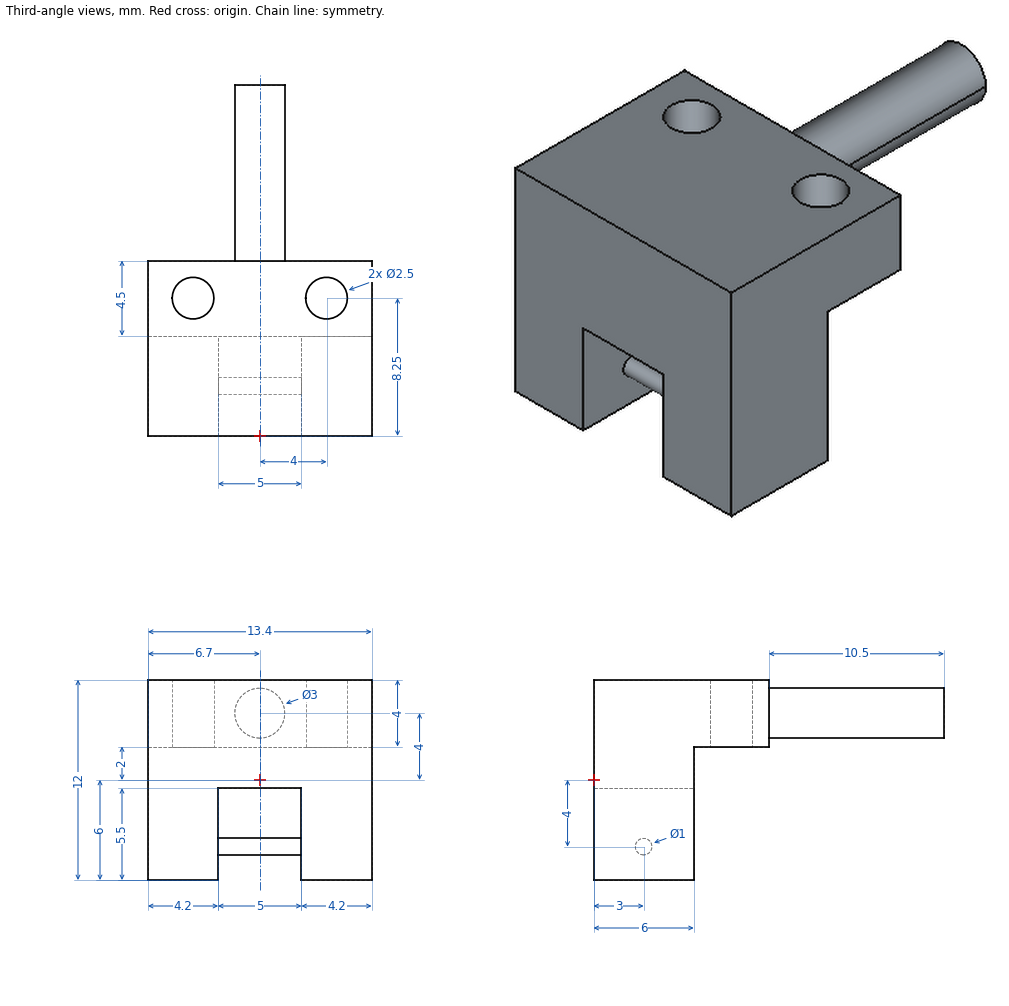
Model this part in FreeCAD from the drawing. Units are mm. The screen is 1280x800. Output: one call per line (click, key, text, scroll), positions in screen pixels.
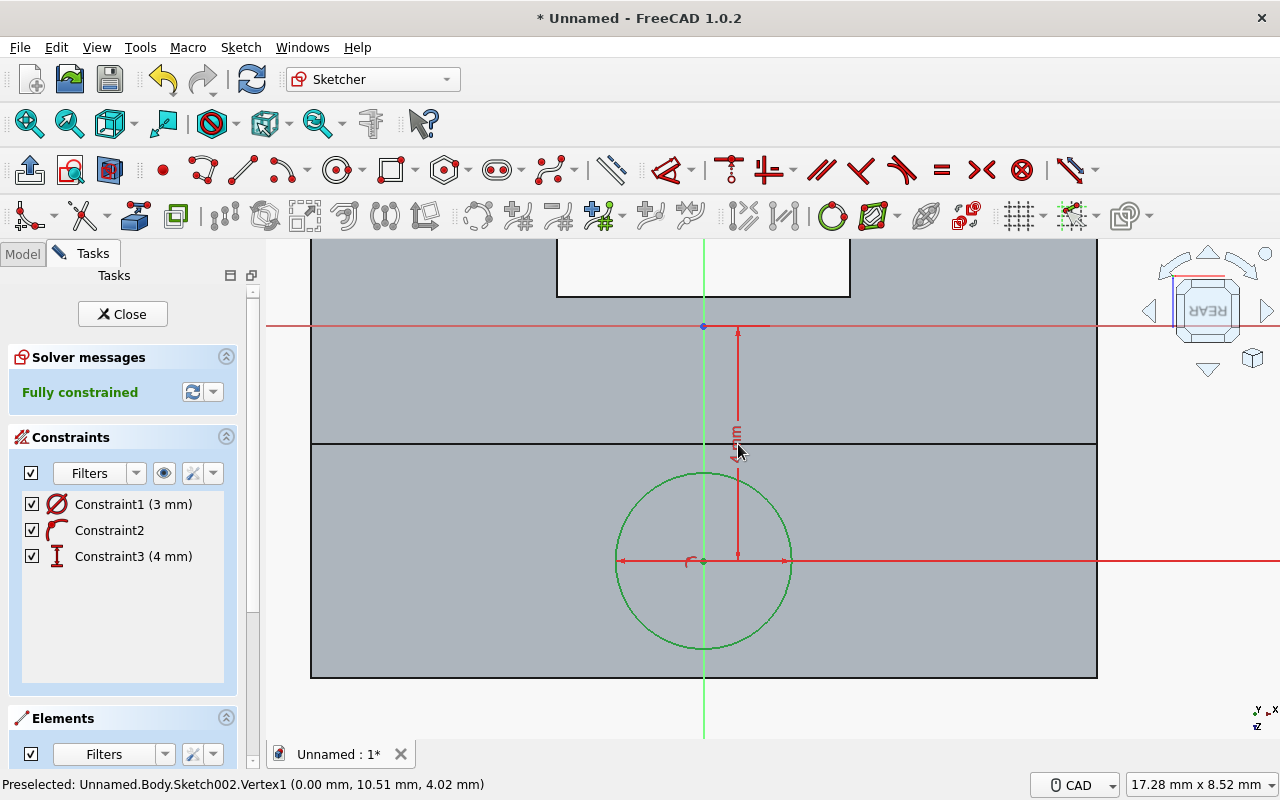
click(123, 314)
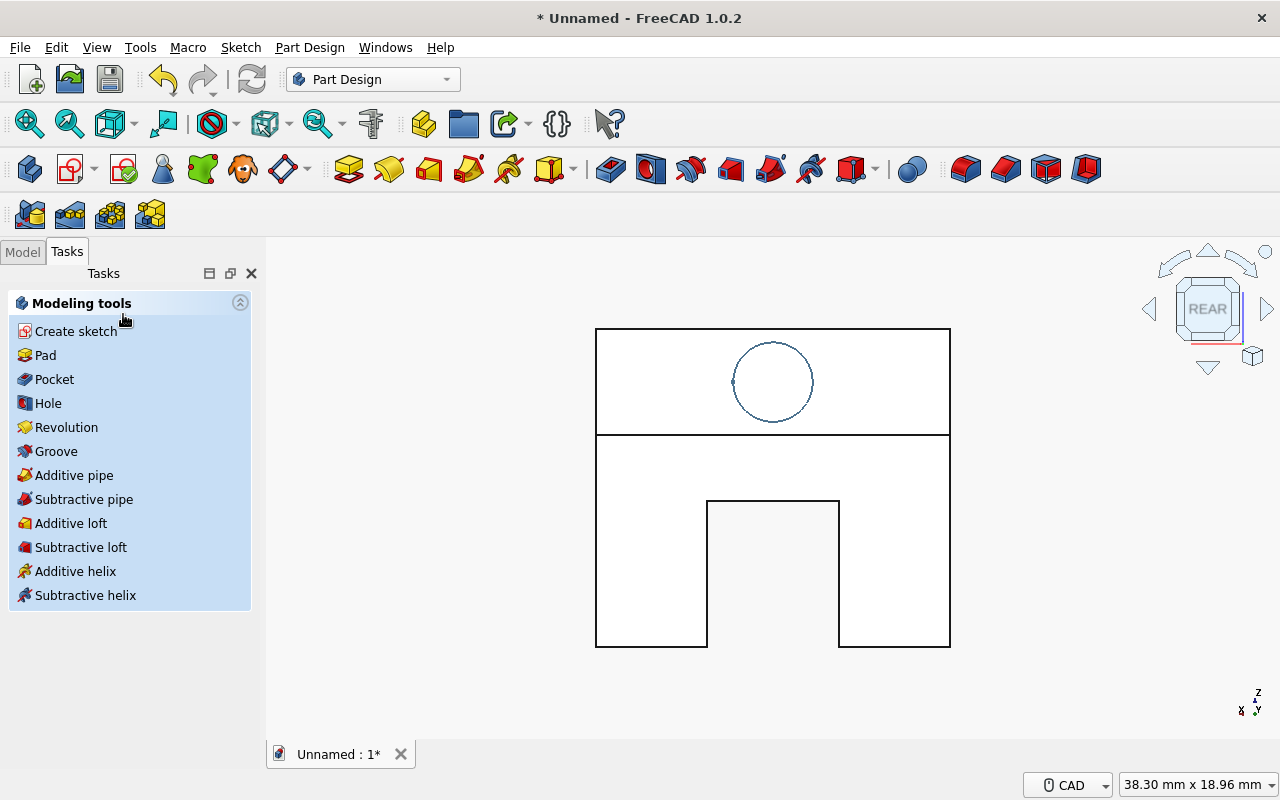
click(350, 170)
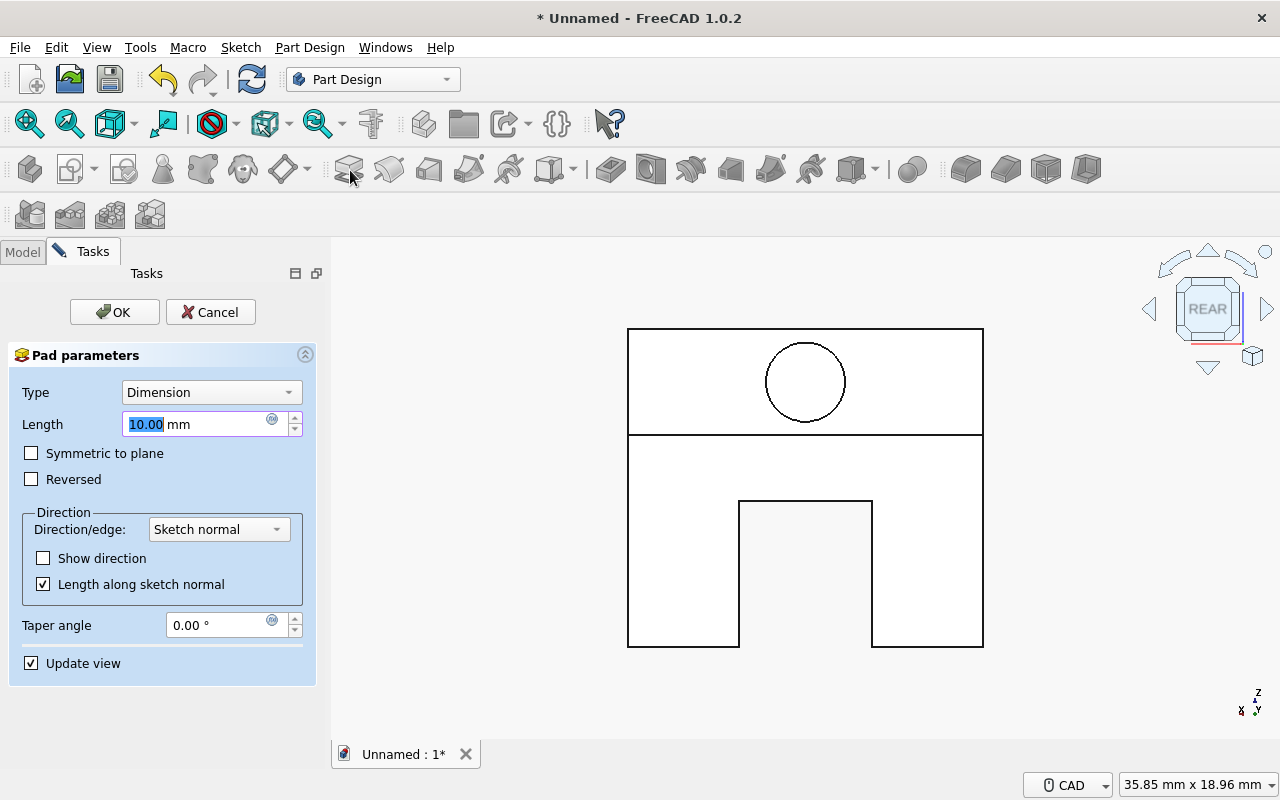
text(10.5)
key(Tab)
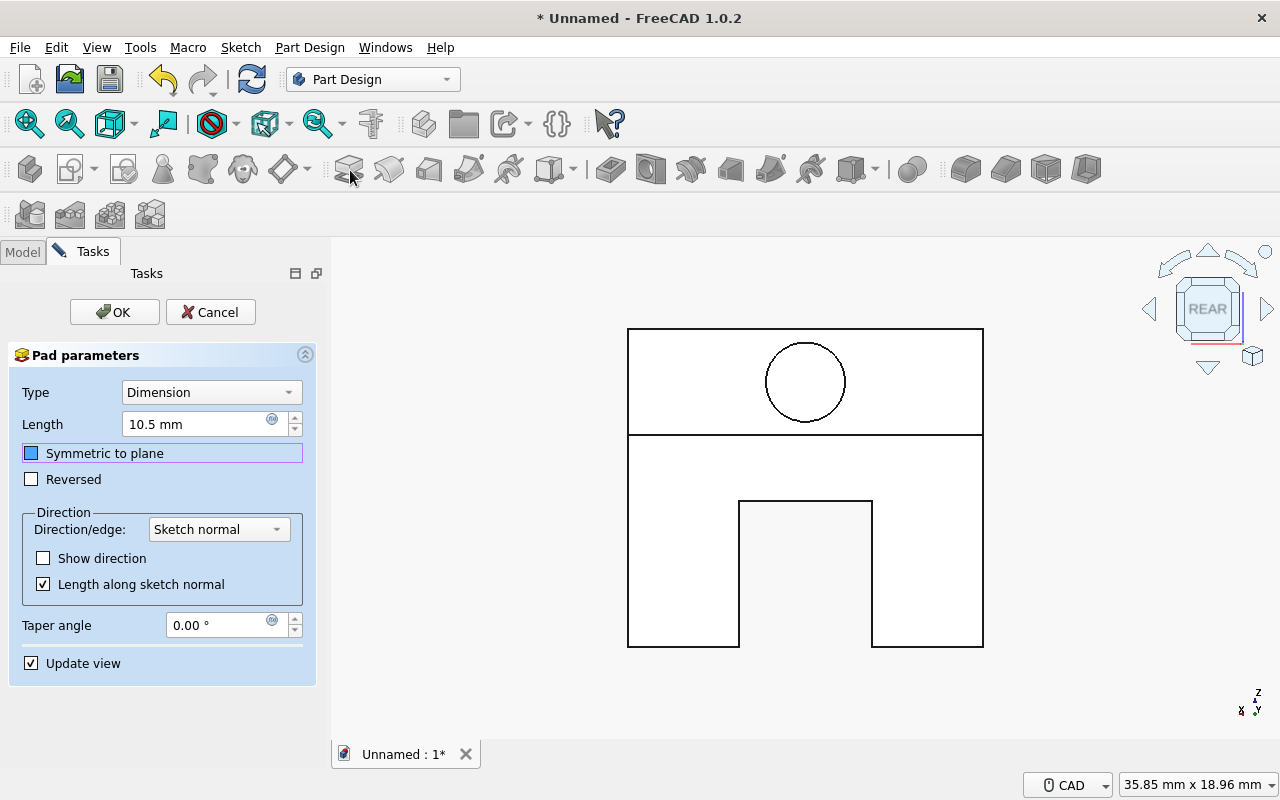
click(115, 312)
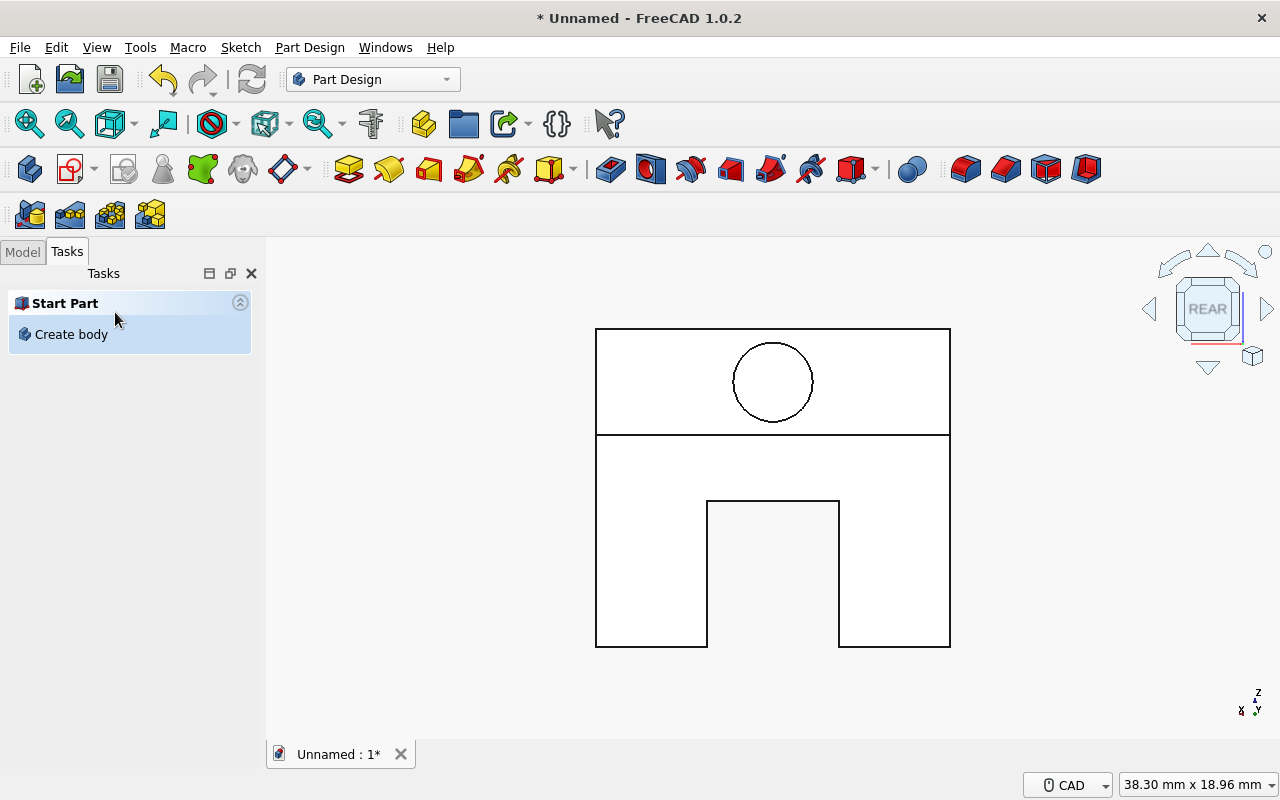
key(5)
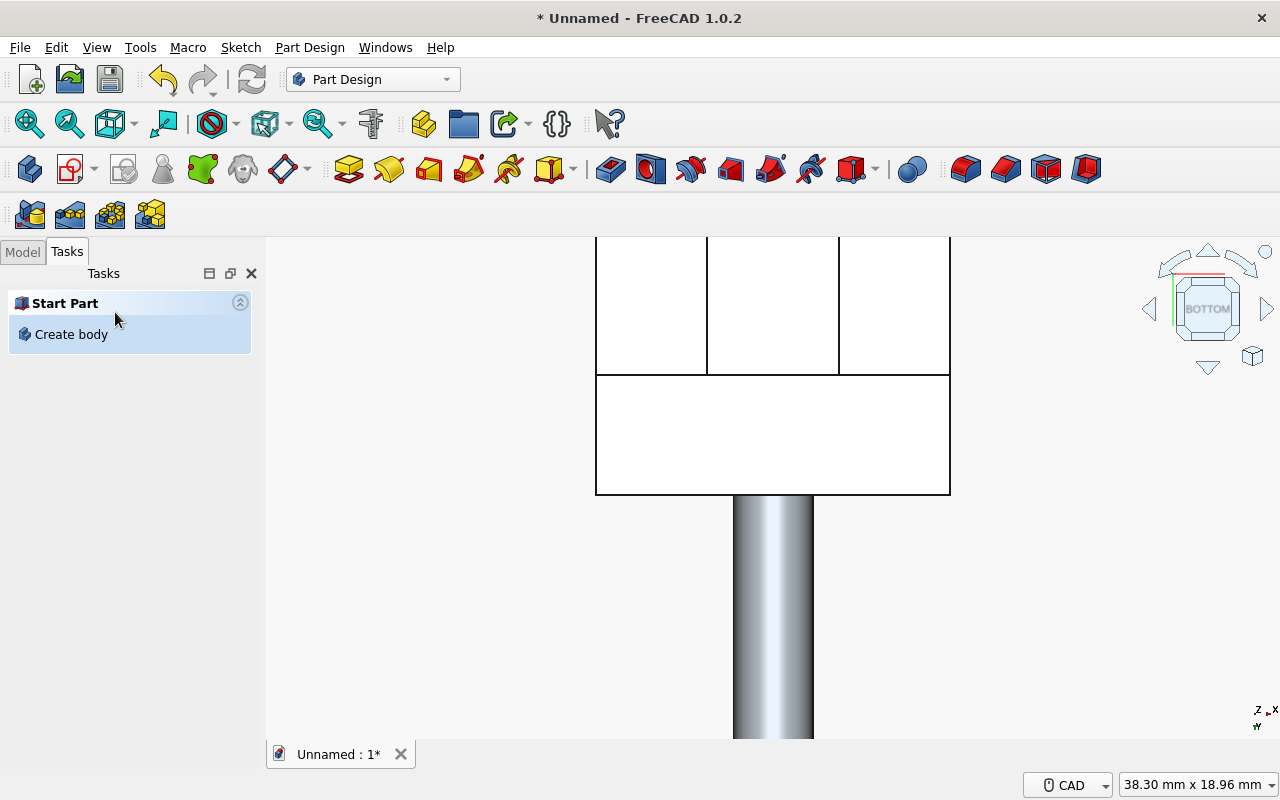
click(30, 124)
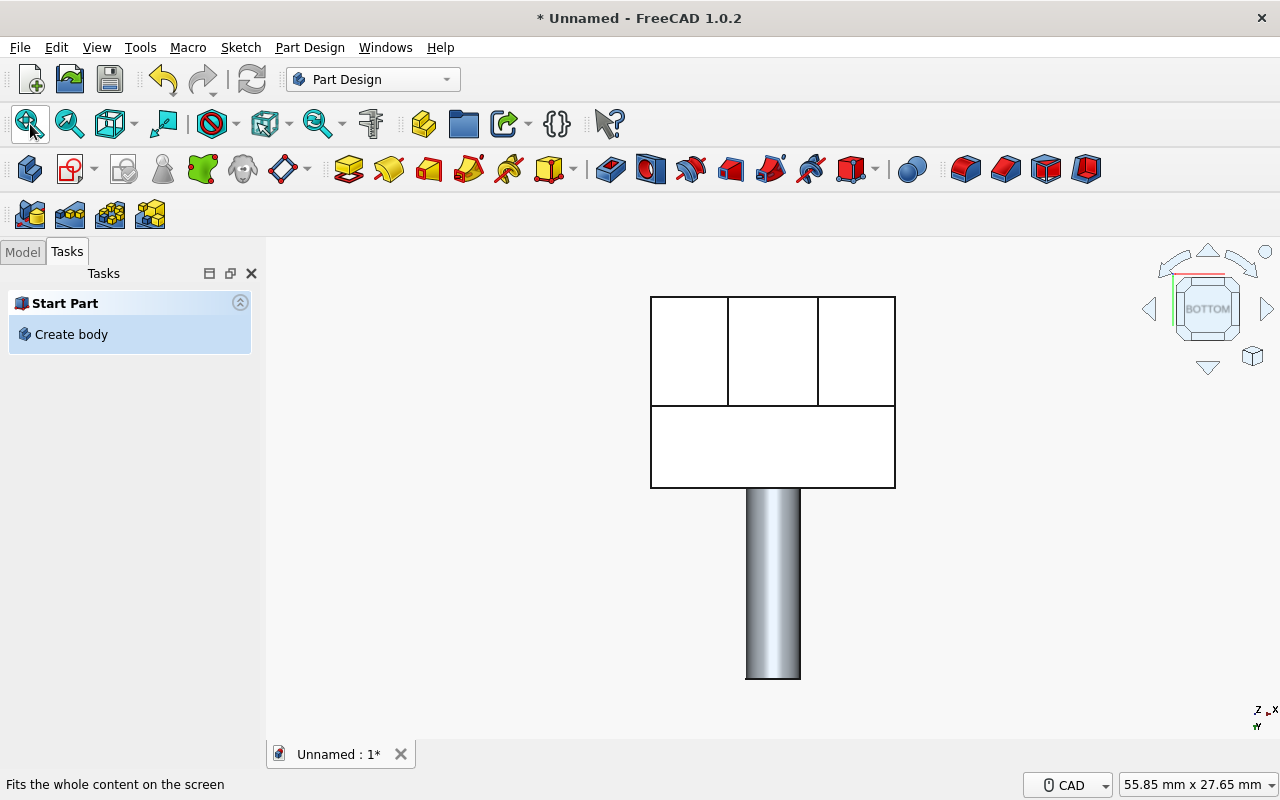
click(843, 446)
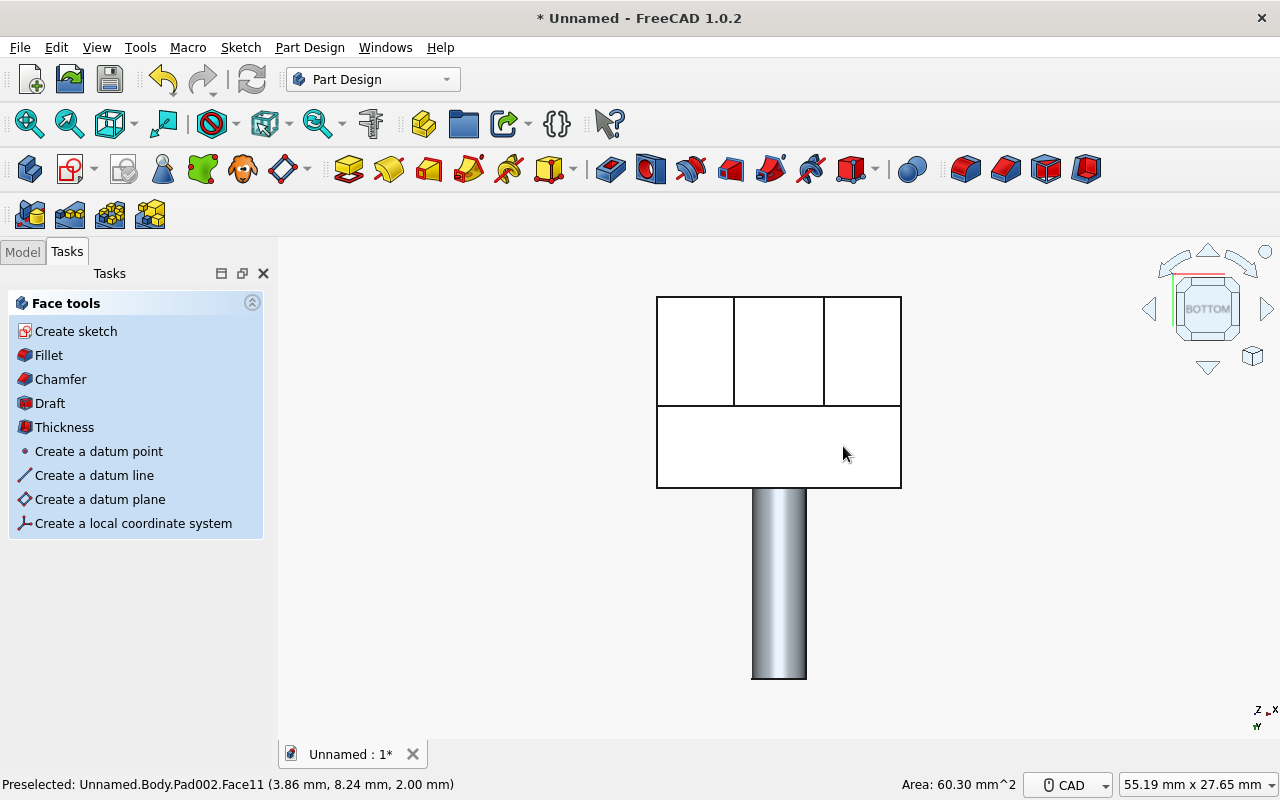
click(70, 170)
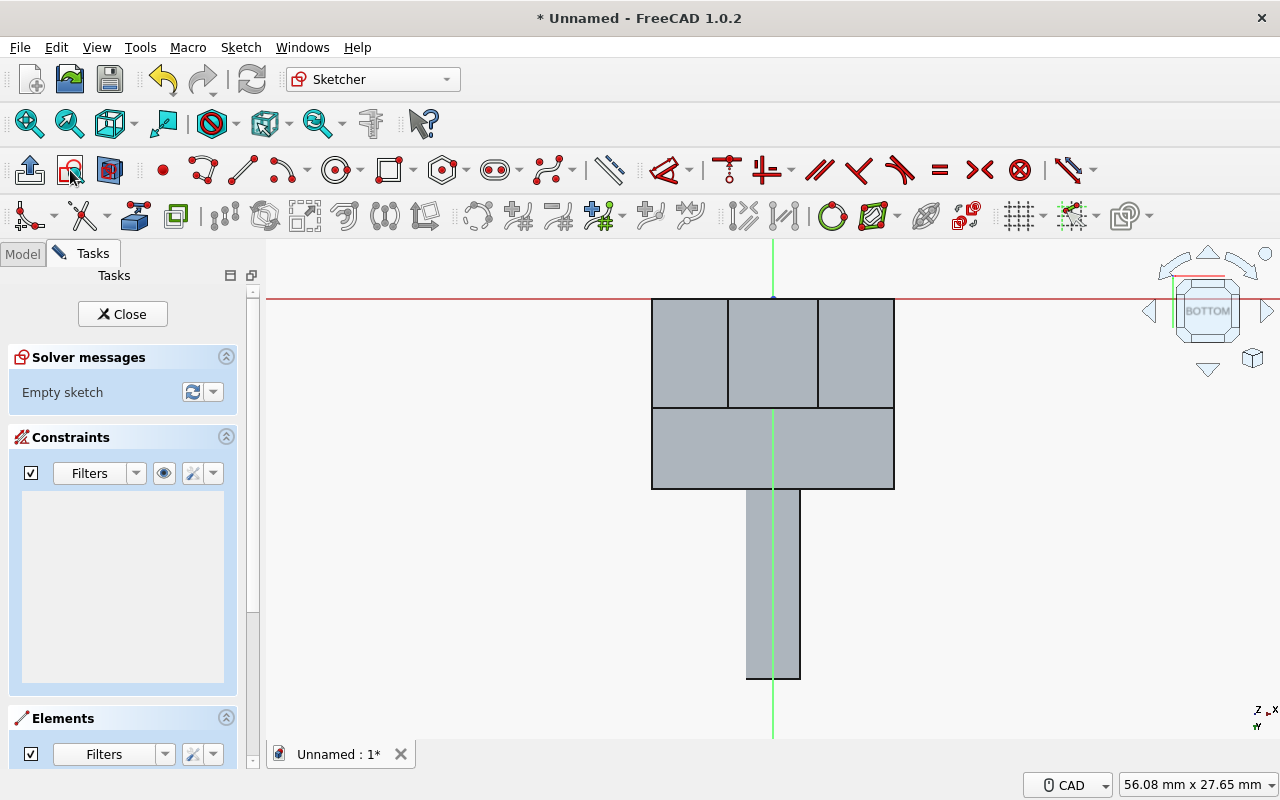
scroll(856, 267, up, 3)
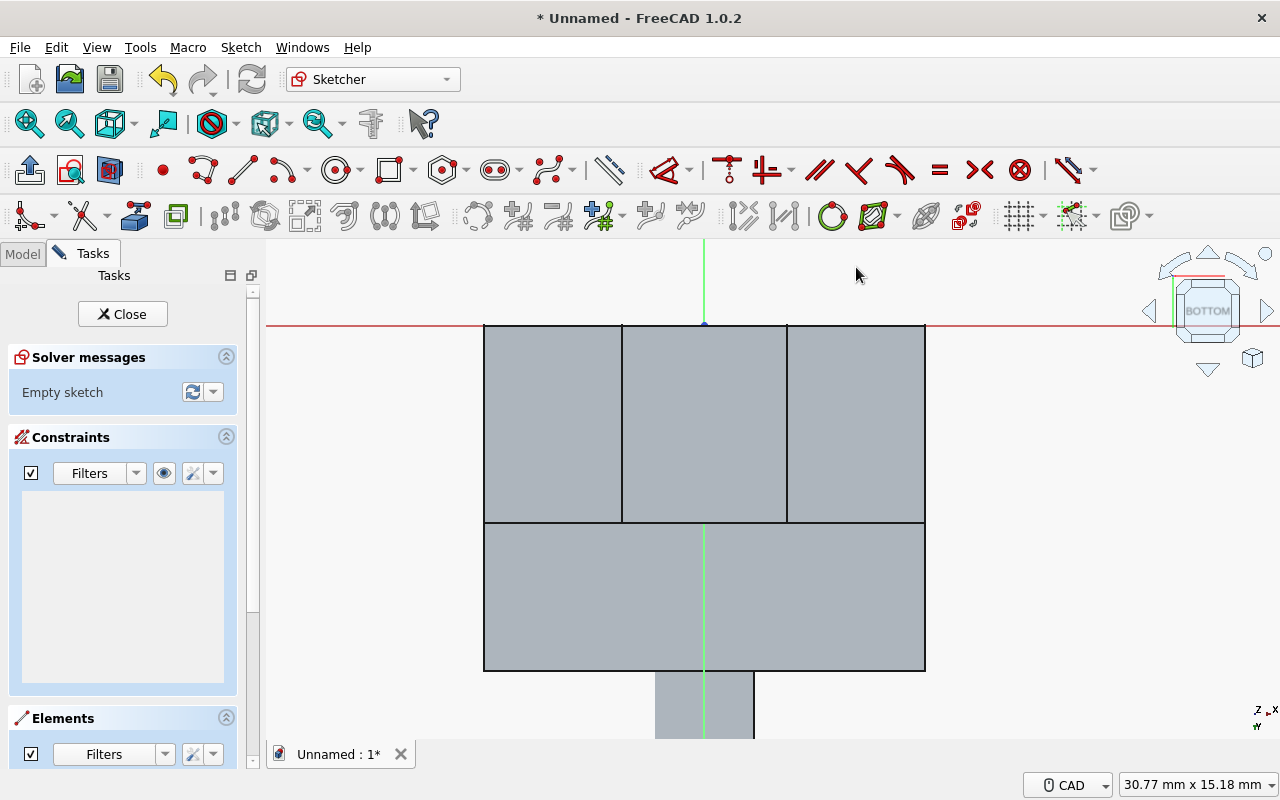
click(336, 170)